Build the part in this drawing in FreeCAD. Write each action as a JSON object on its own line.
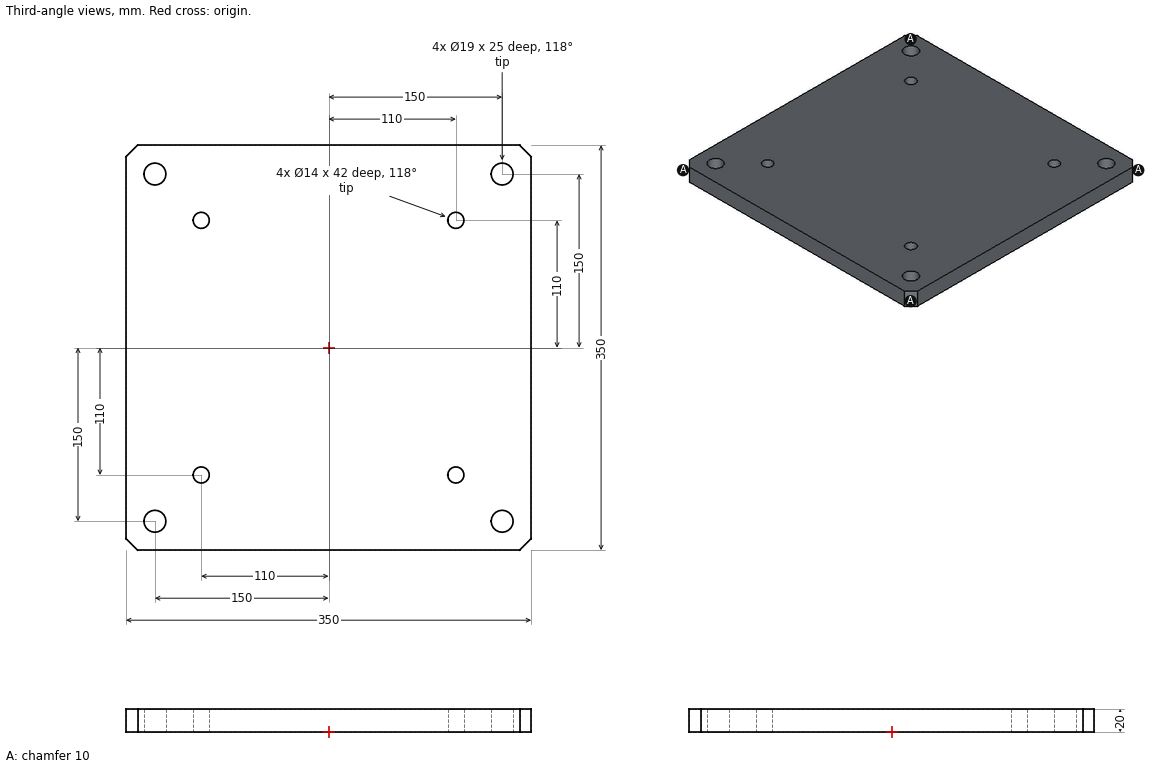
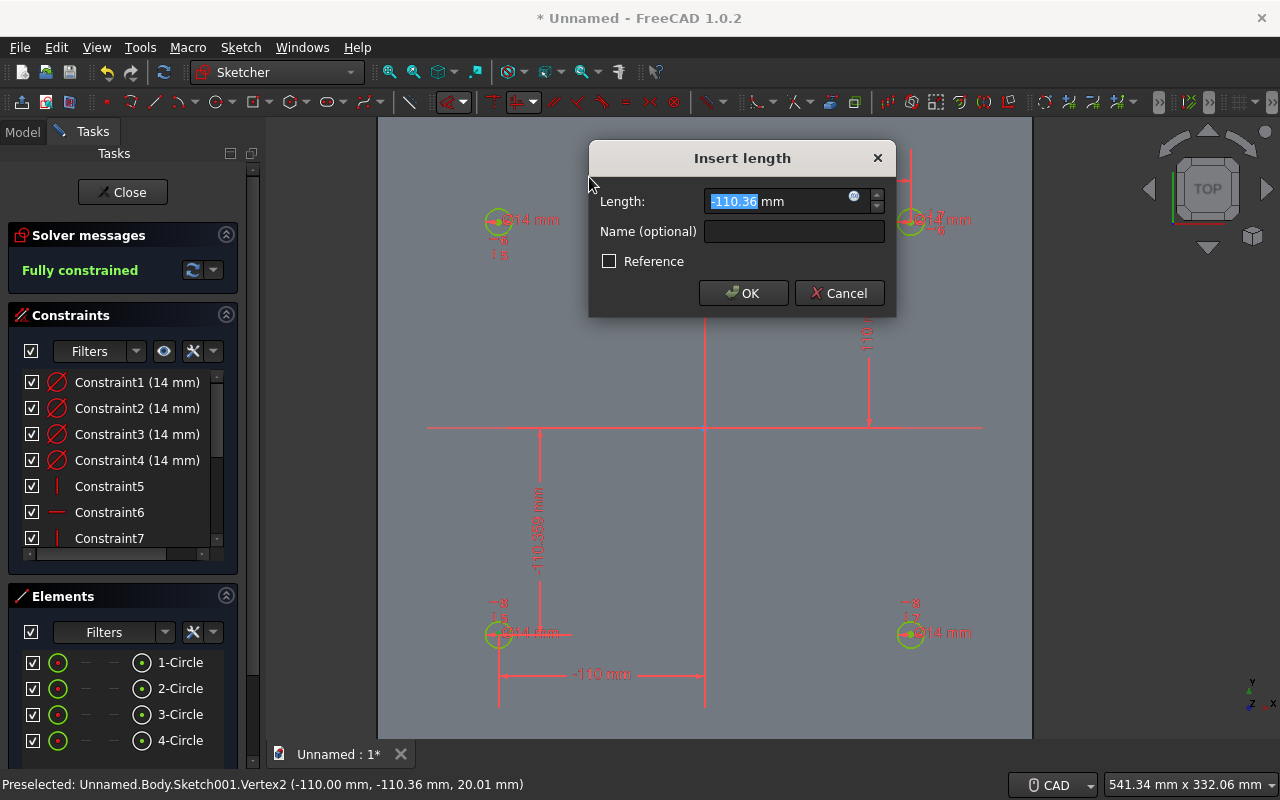
{"action": "type", "text": "-110"}
{"action": "key", "text": "Return"}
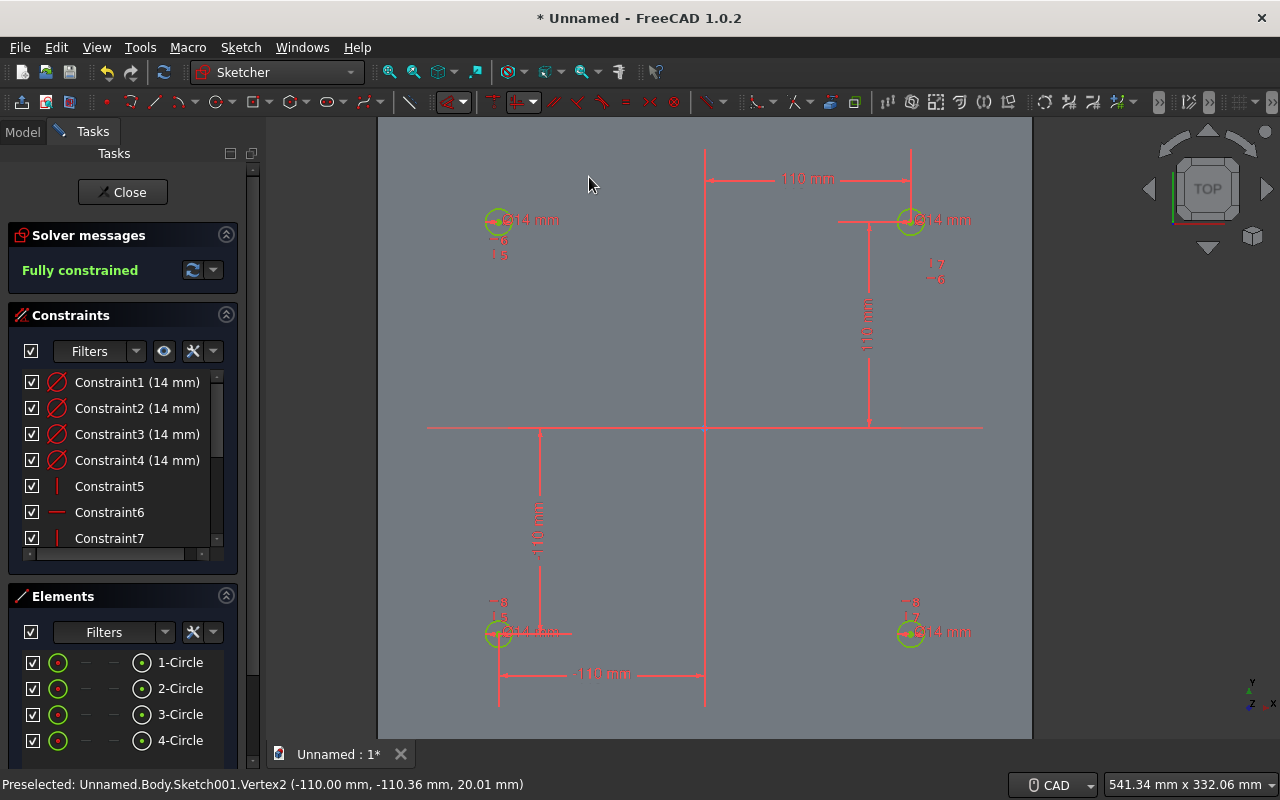
{"action": "left_click", "coordinate": [123, 192]}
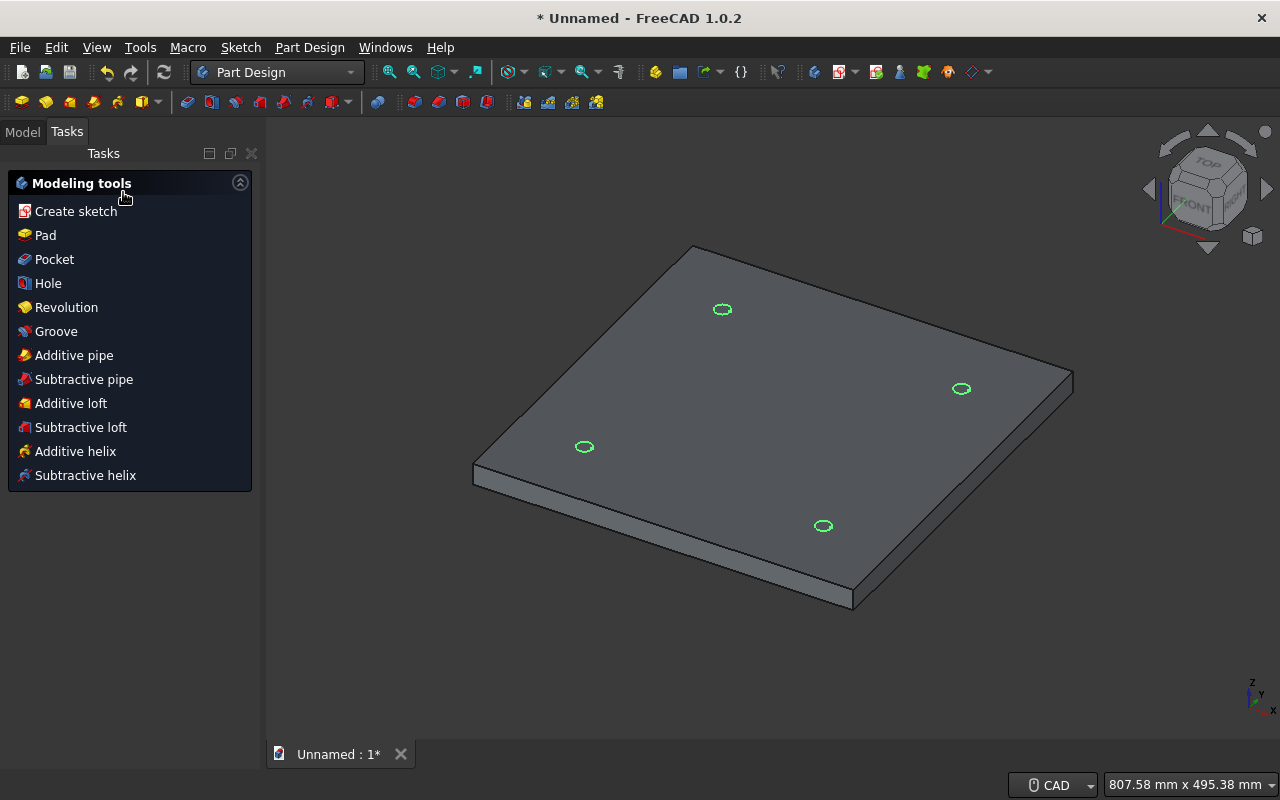
{"action": "left_click", "coordinate": [212, 102]}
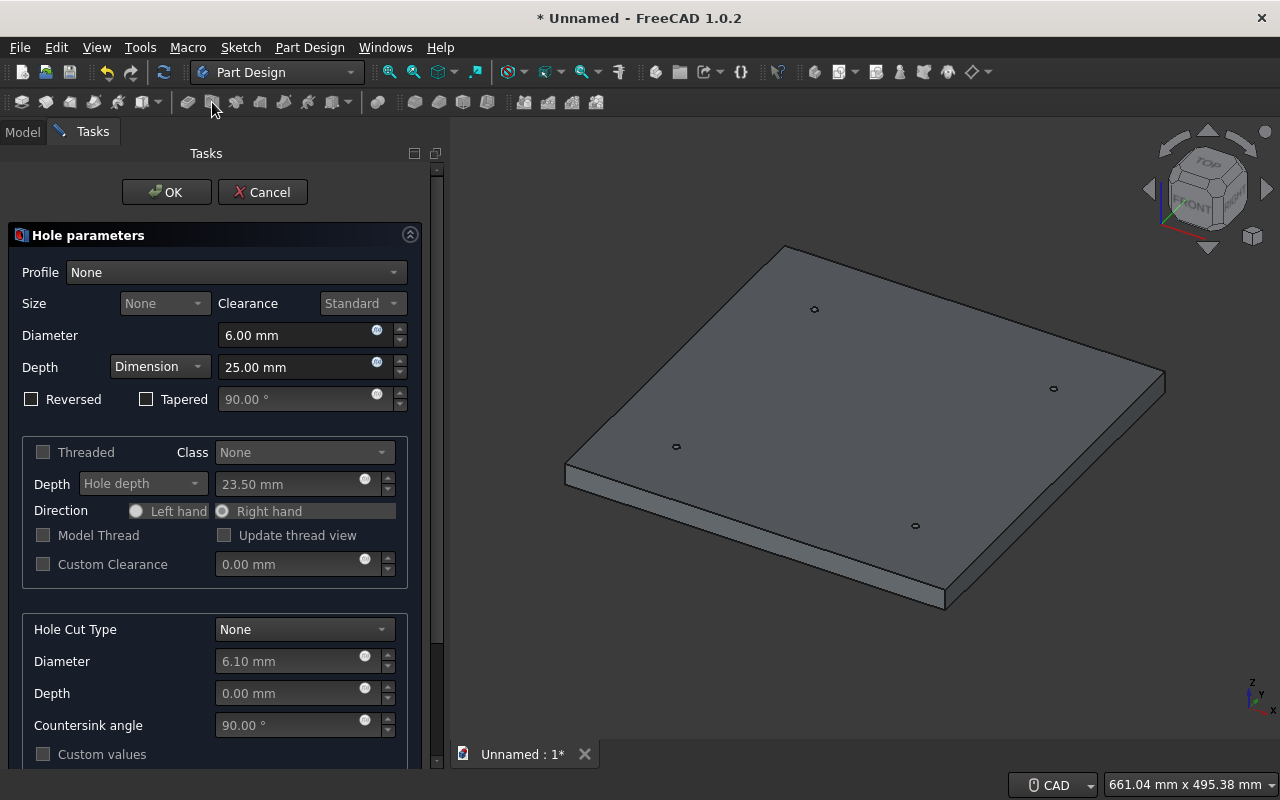
{"action": "triple_click", "coordinate": [305, 335]}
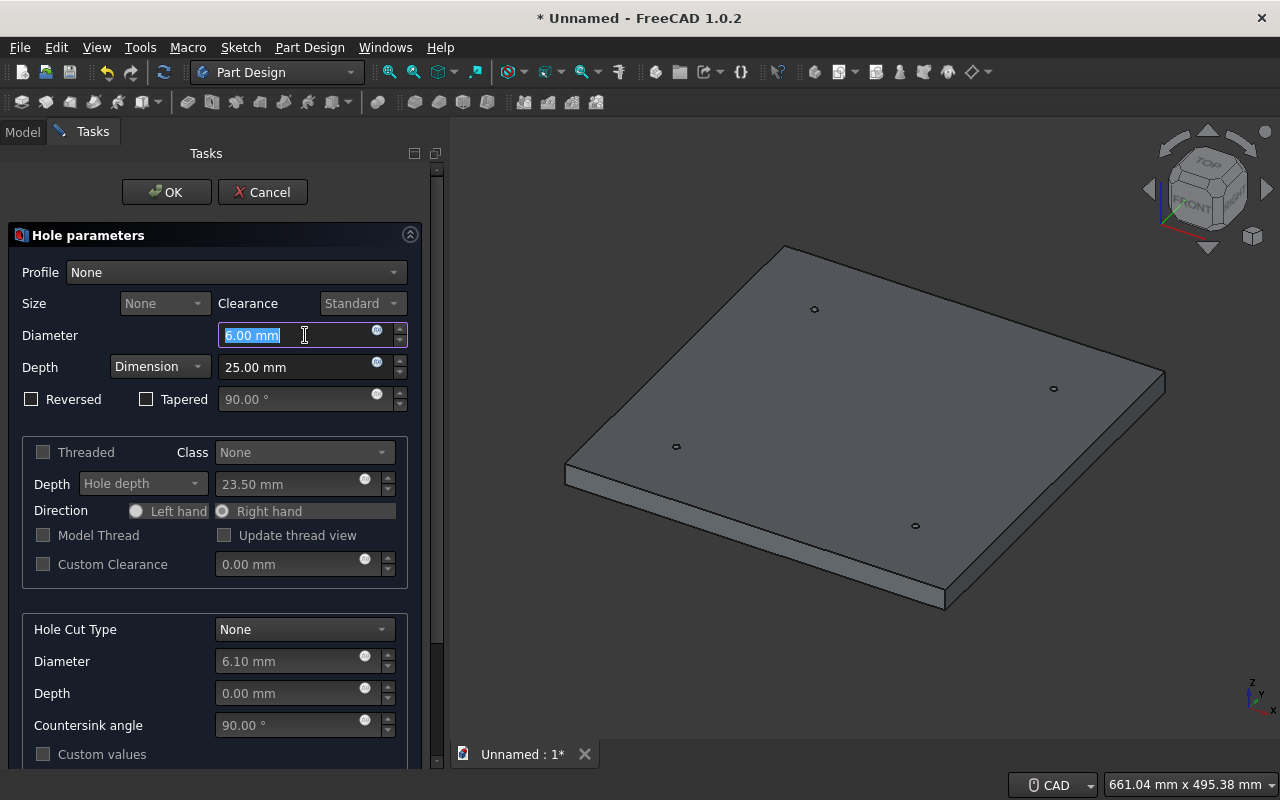
{"action": "type", "text": "14"}
{"action": "key", "text": "Tab"}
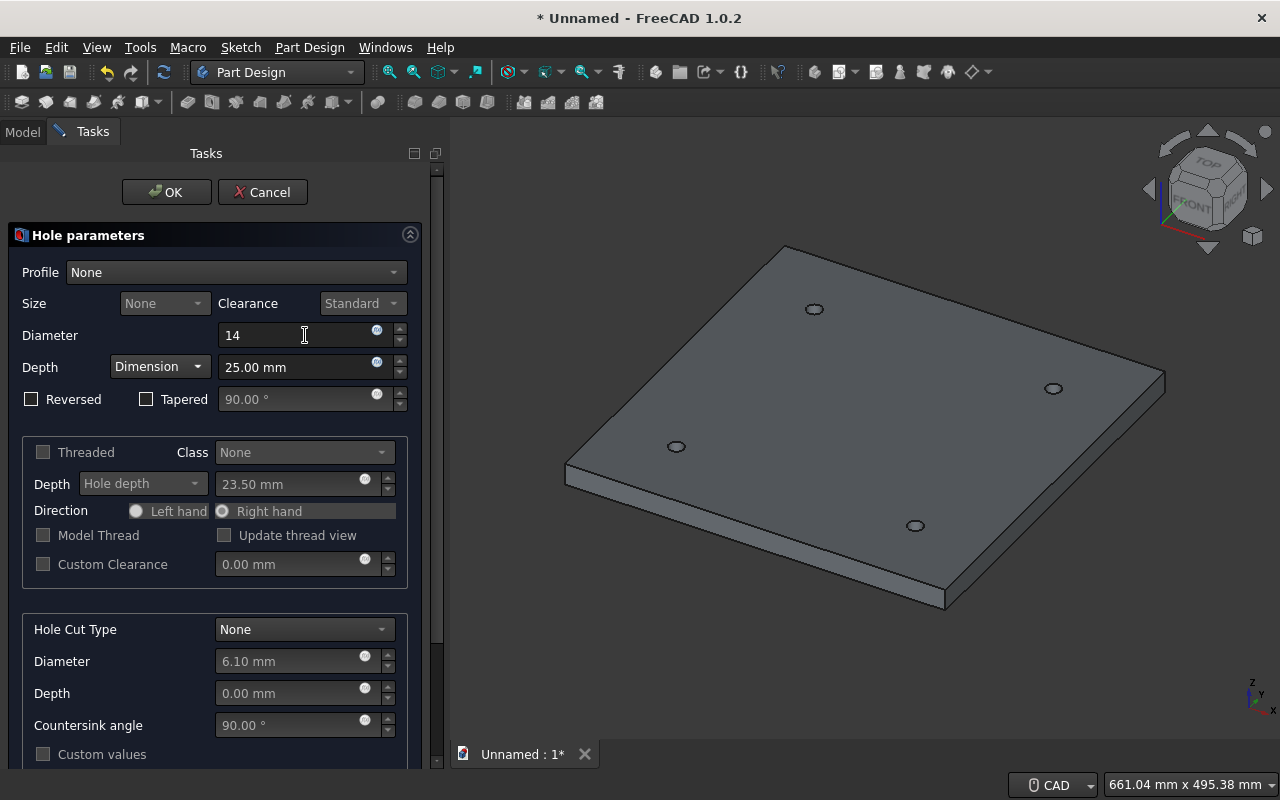
{"action": "triple_click", "coordinate": [305, 367]}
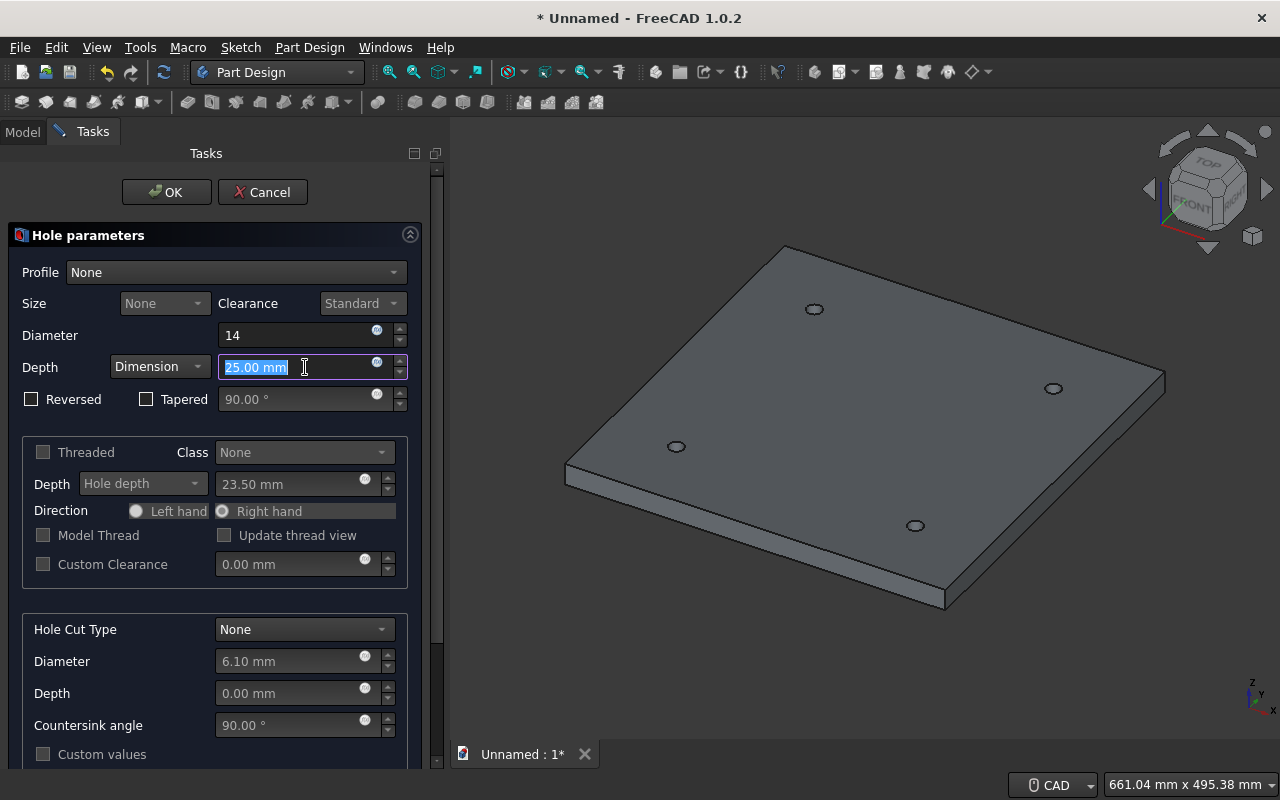
{"action": "type", "text": "42"}
{"action": "key", "text": "Tab"}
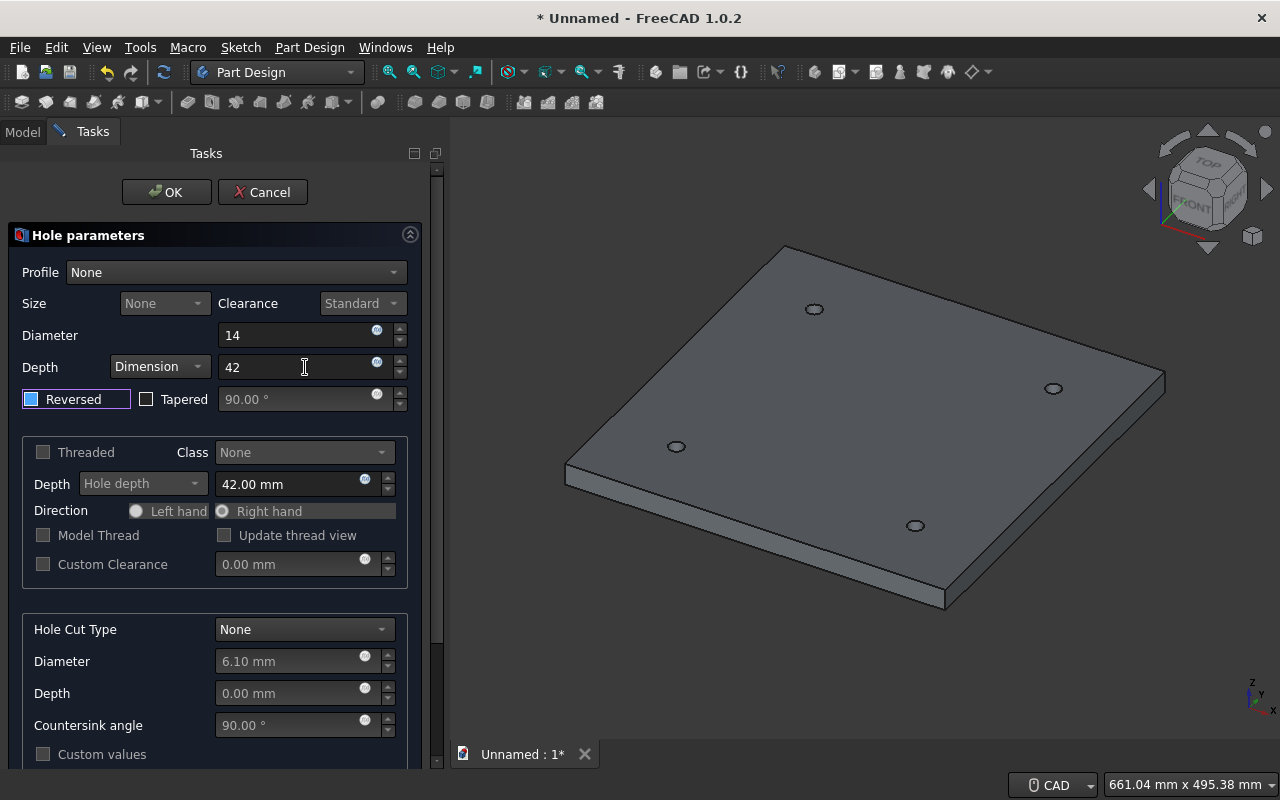
{"action": "left_click", "coordinate": [167, 192]}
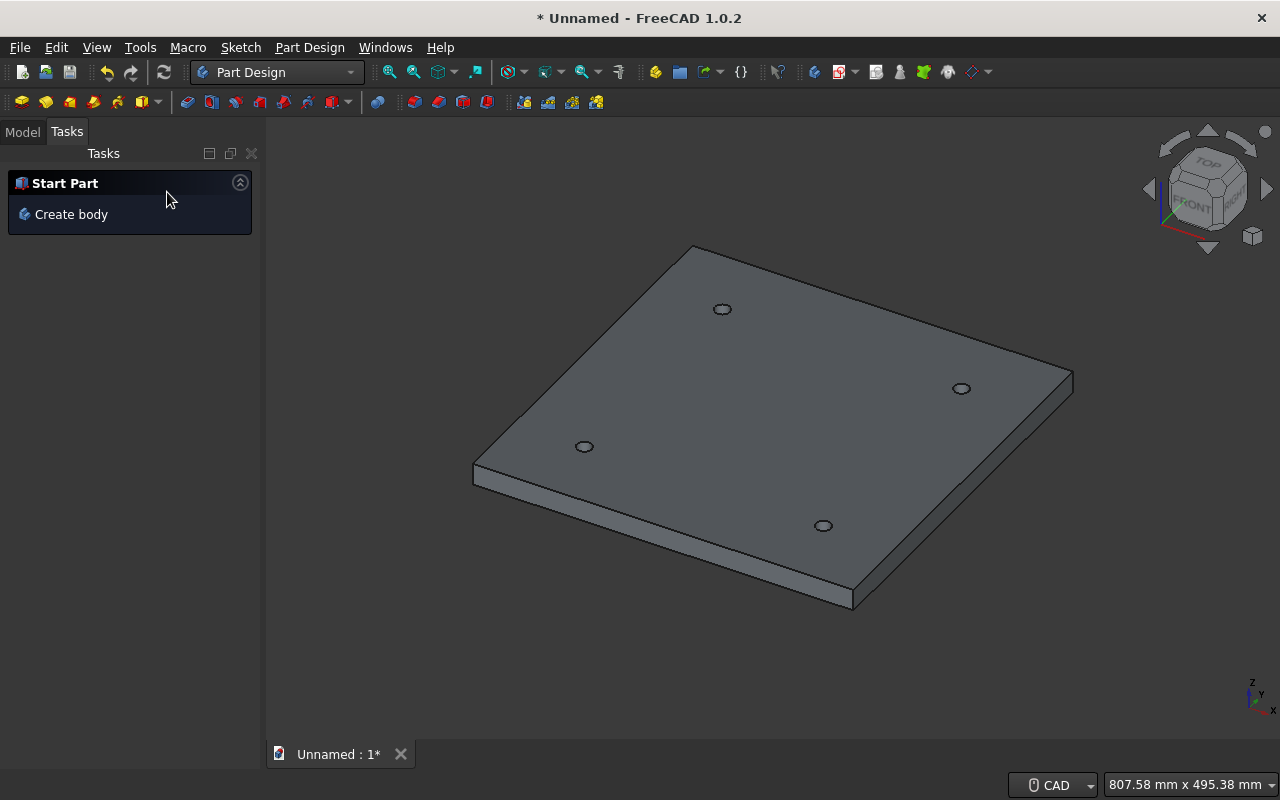
{"action": "left_click", "coordinate": [773, 417]}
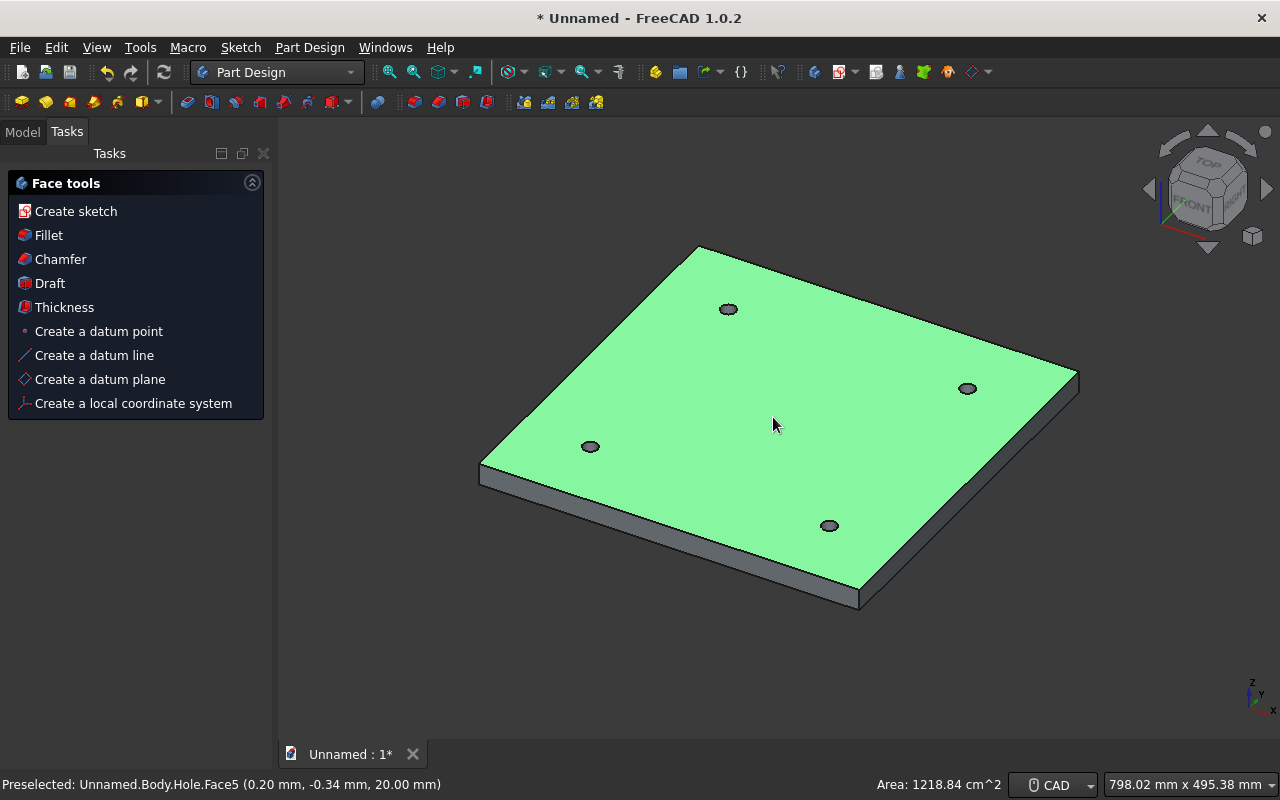
{"action": "left_click", "coordinate": [840, 72]}